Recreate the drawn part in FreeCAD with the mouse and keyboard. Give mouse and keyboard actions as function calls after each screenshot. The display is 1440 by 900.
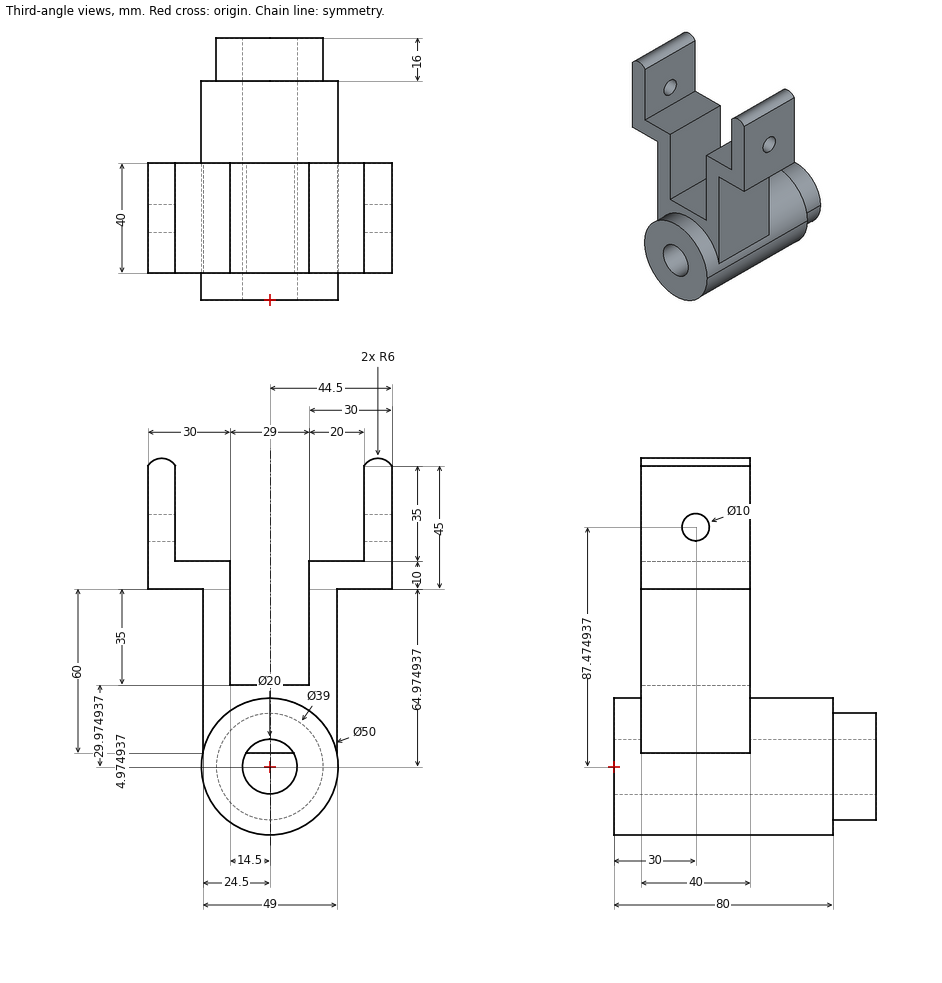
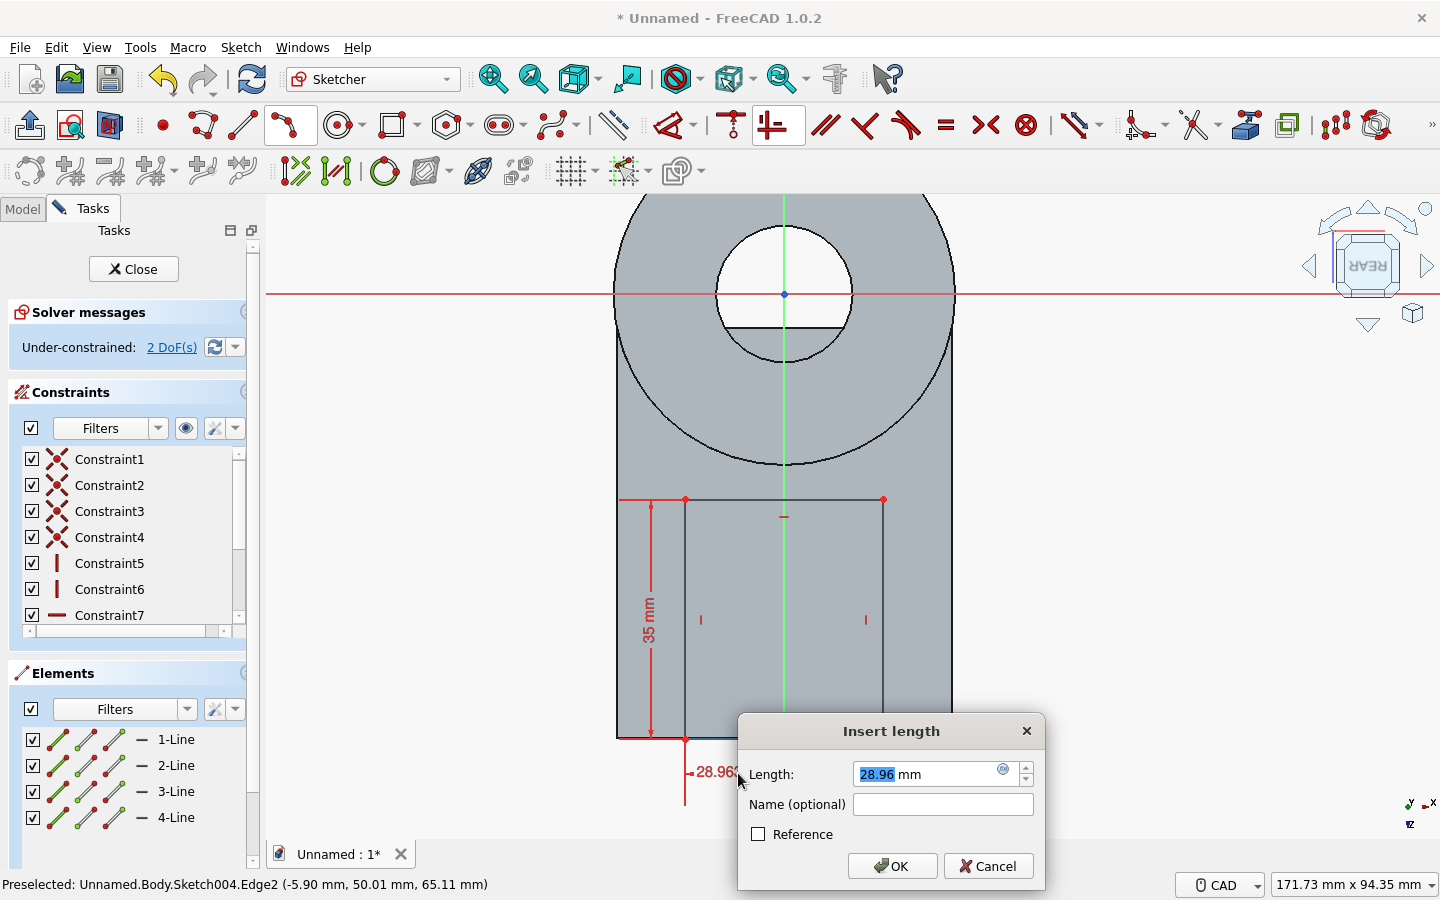
text(29)
key(Return)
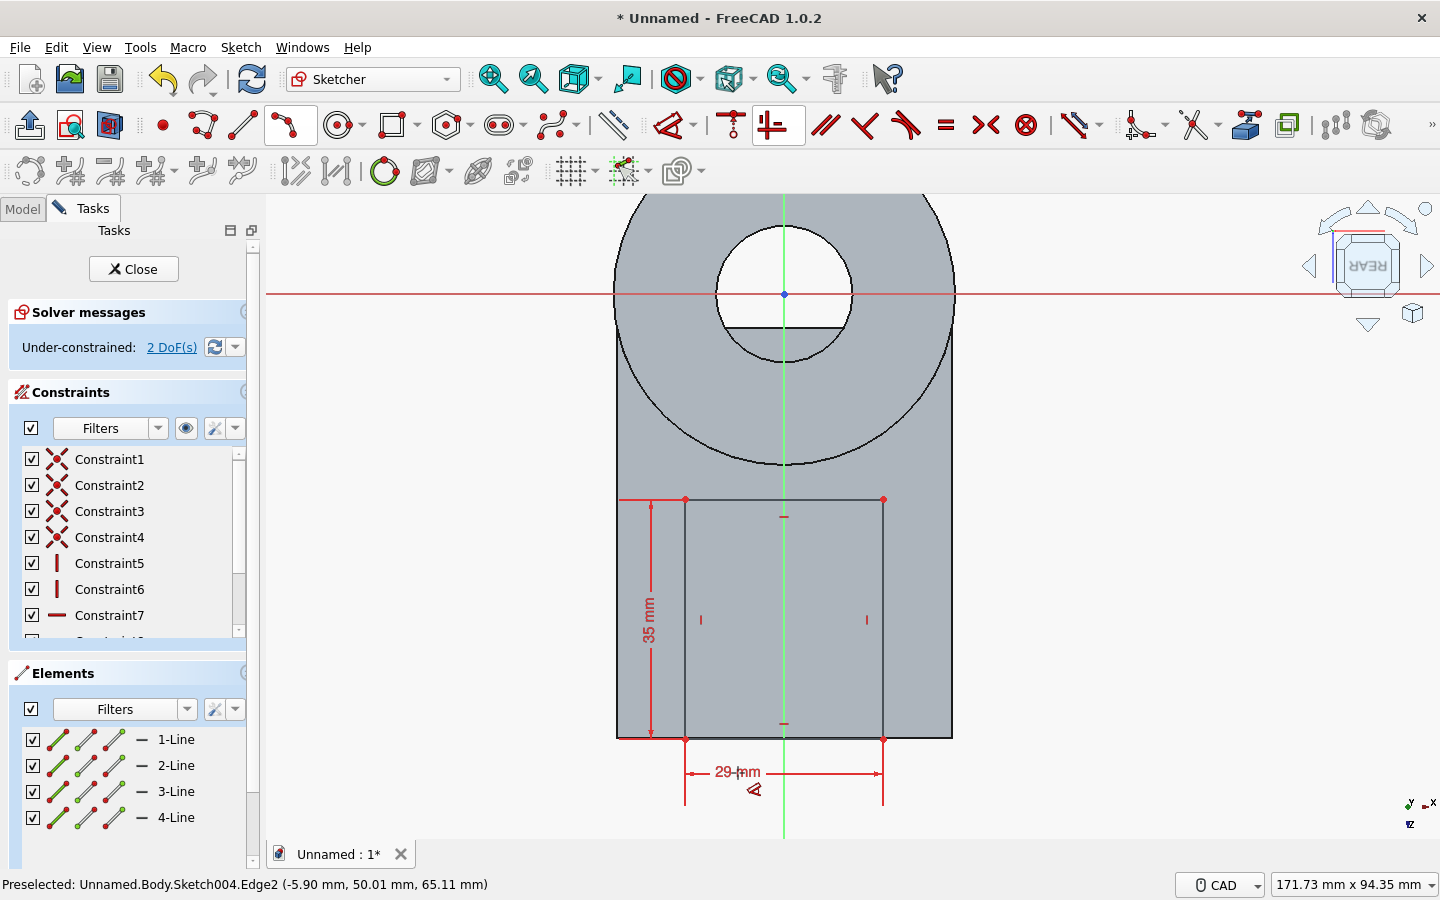
click(685, 500)
click(735, 260)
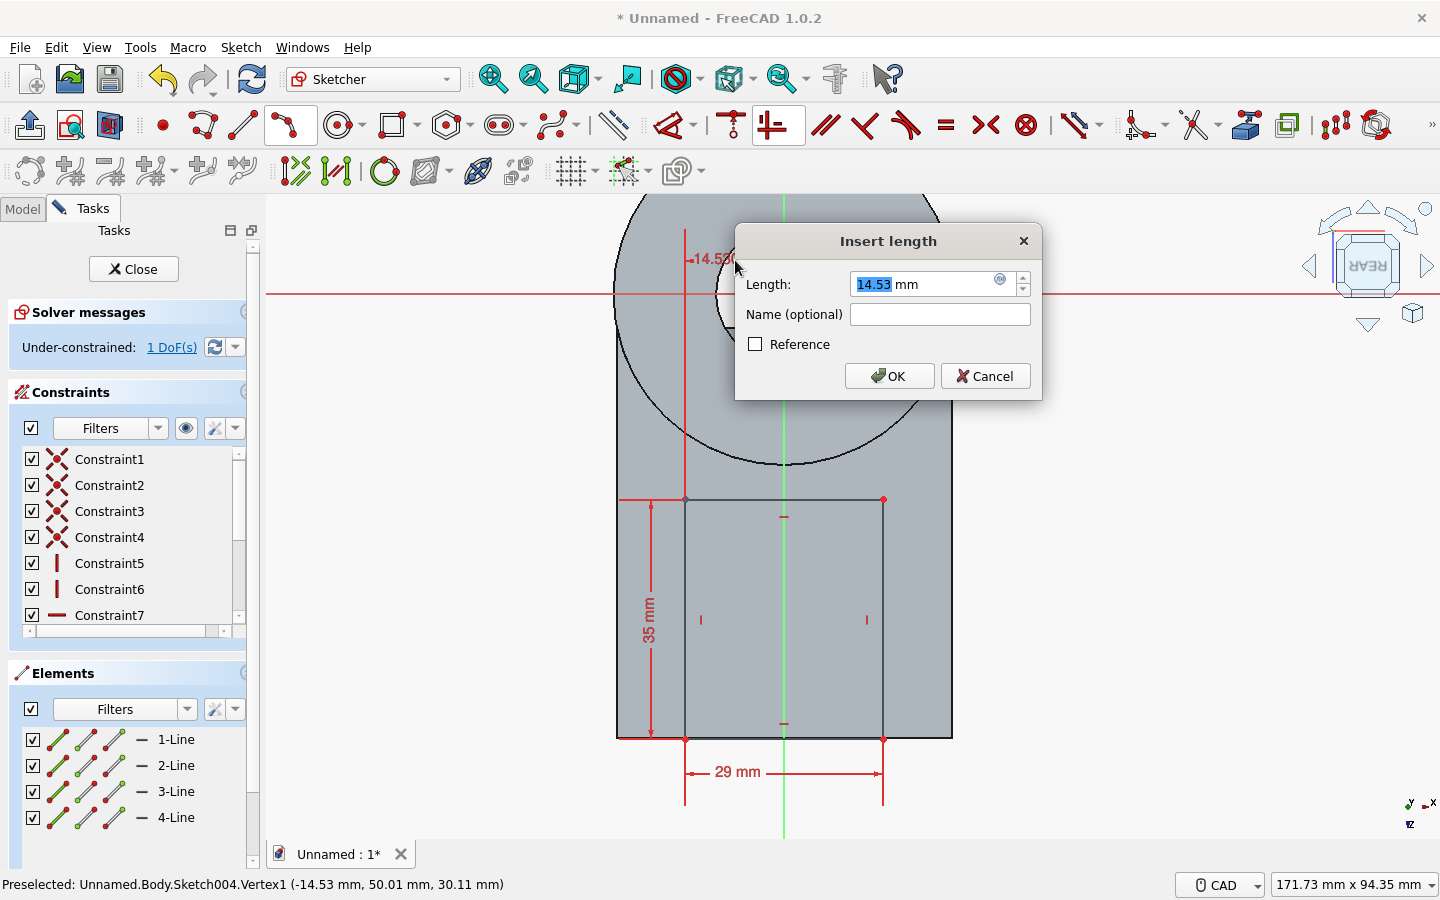
text(14.5)
key(Return)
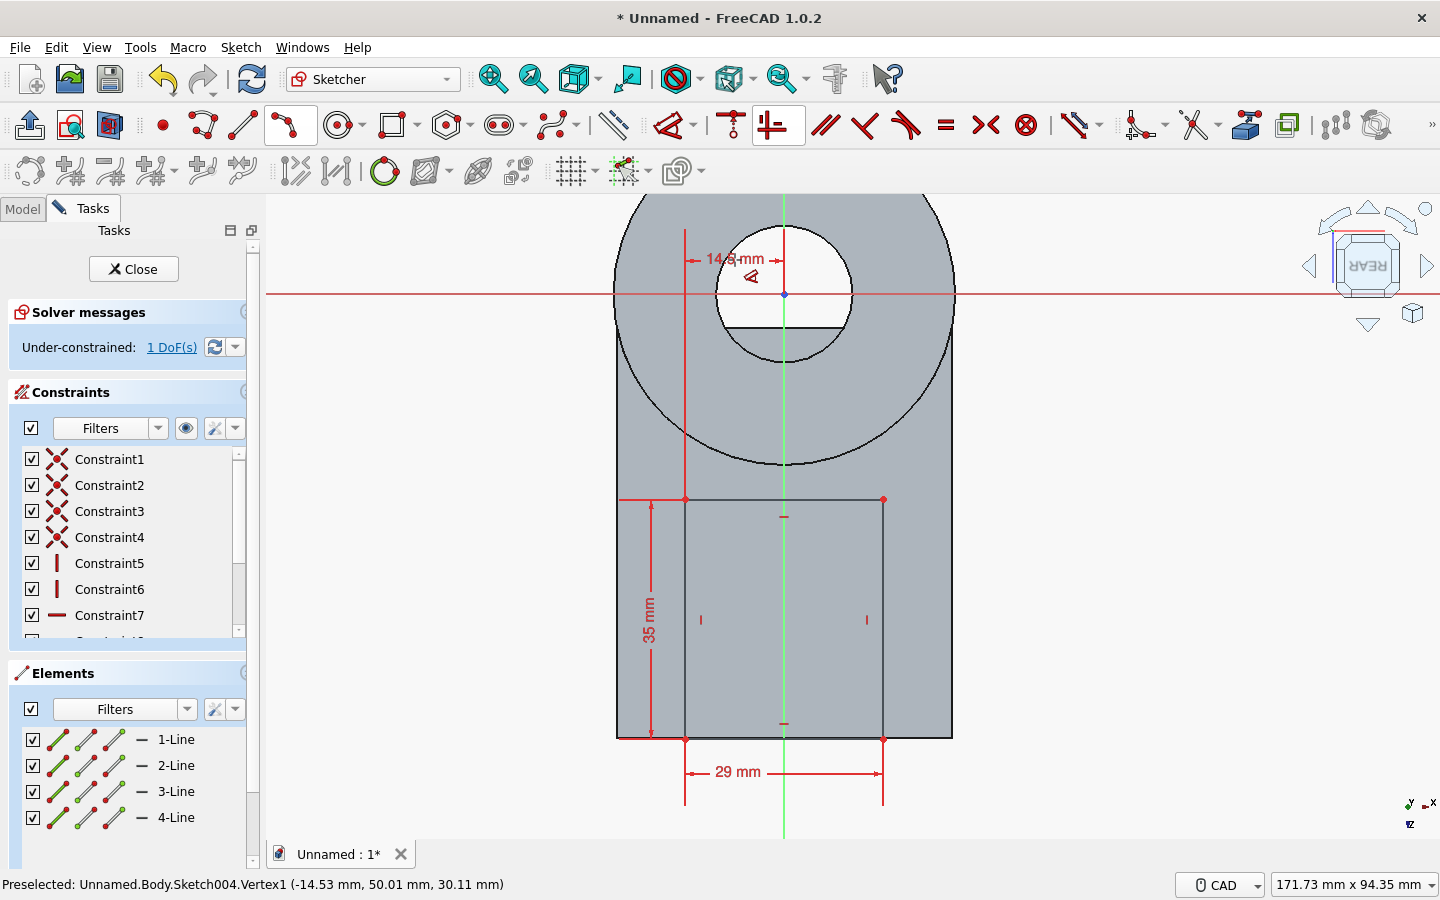
click(685, 500)
click(651, 397)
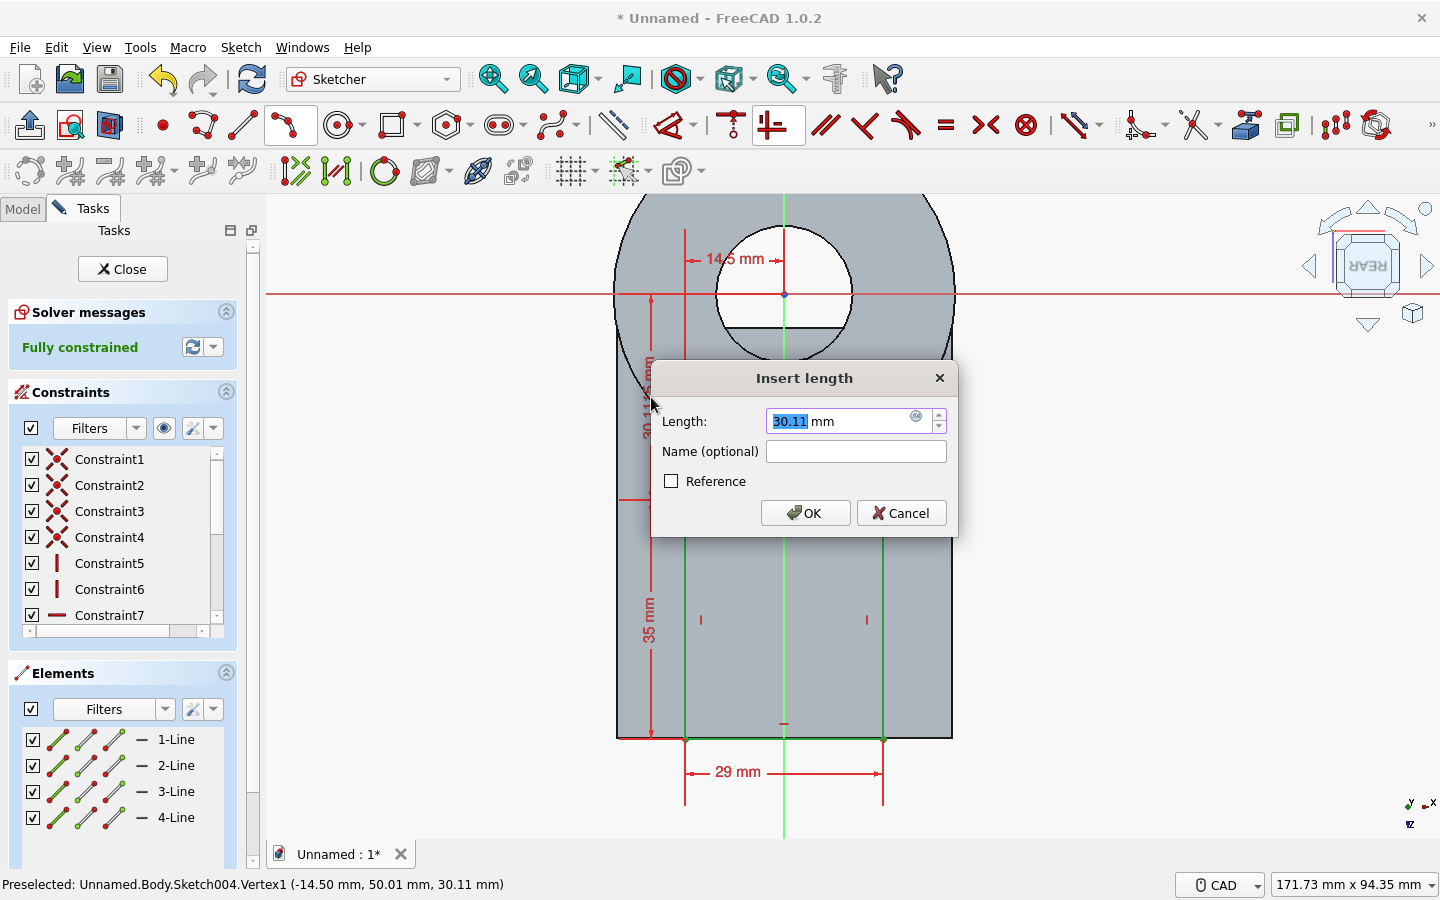
text(29.974937)
key(Return)
key(Escape)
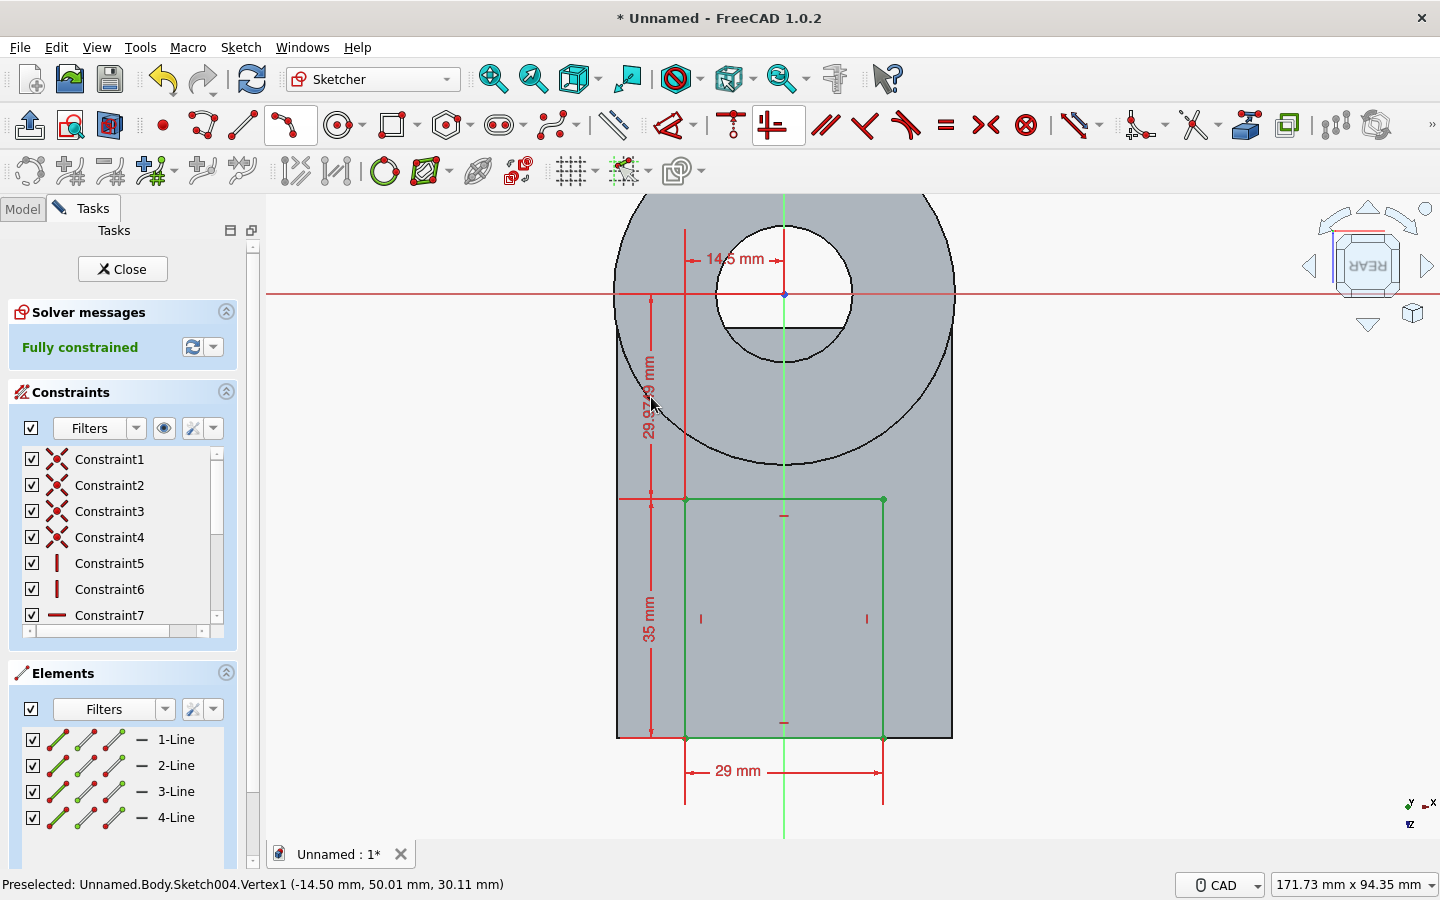
click(123, 269)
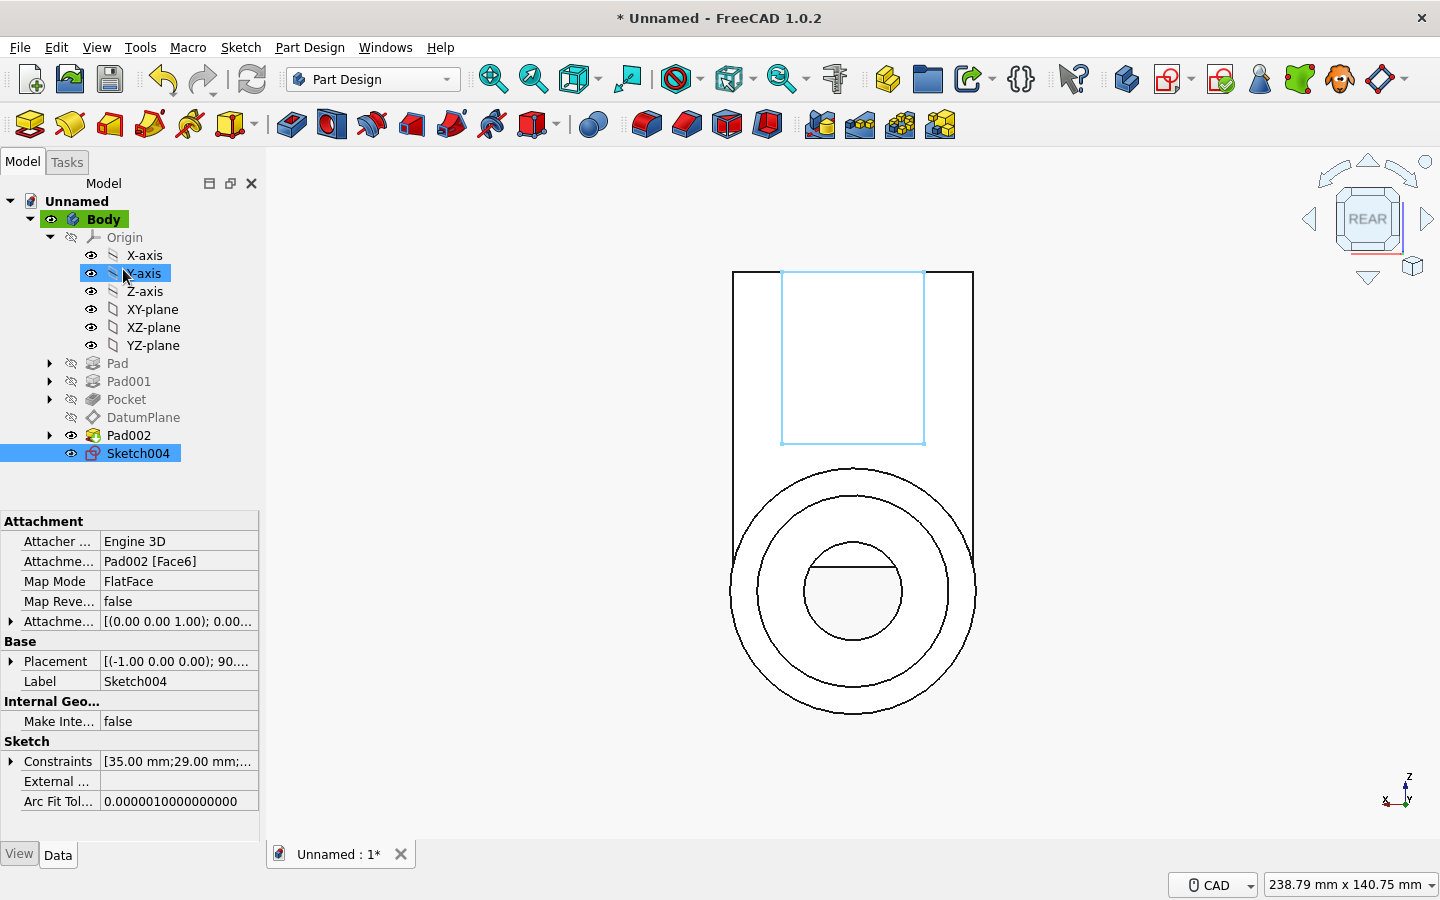
click(292, 124)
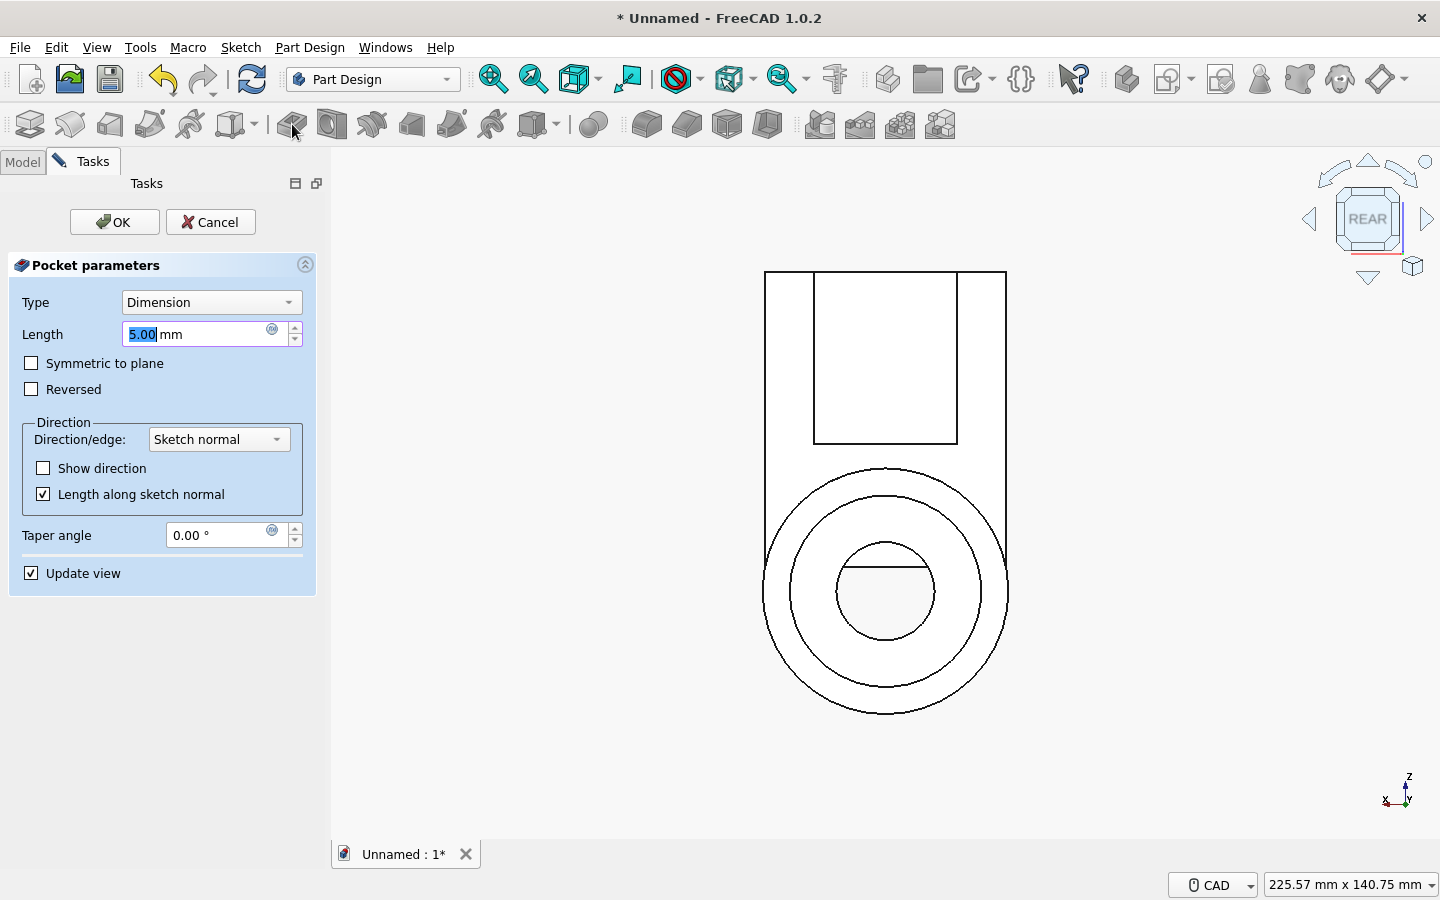
text(40)
key(Tab)